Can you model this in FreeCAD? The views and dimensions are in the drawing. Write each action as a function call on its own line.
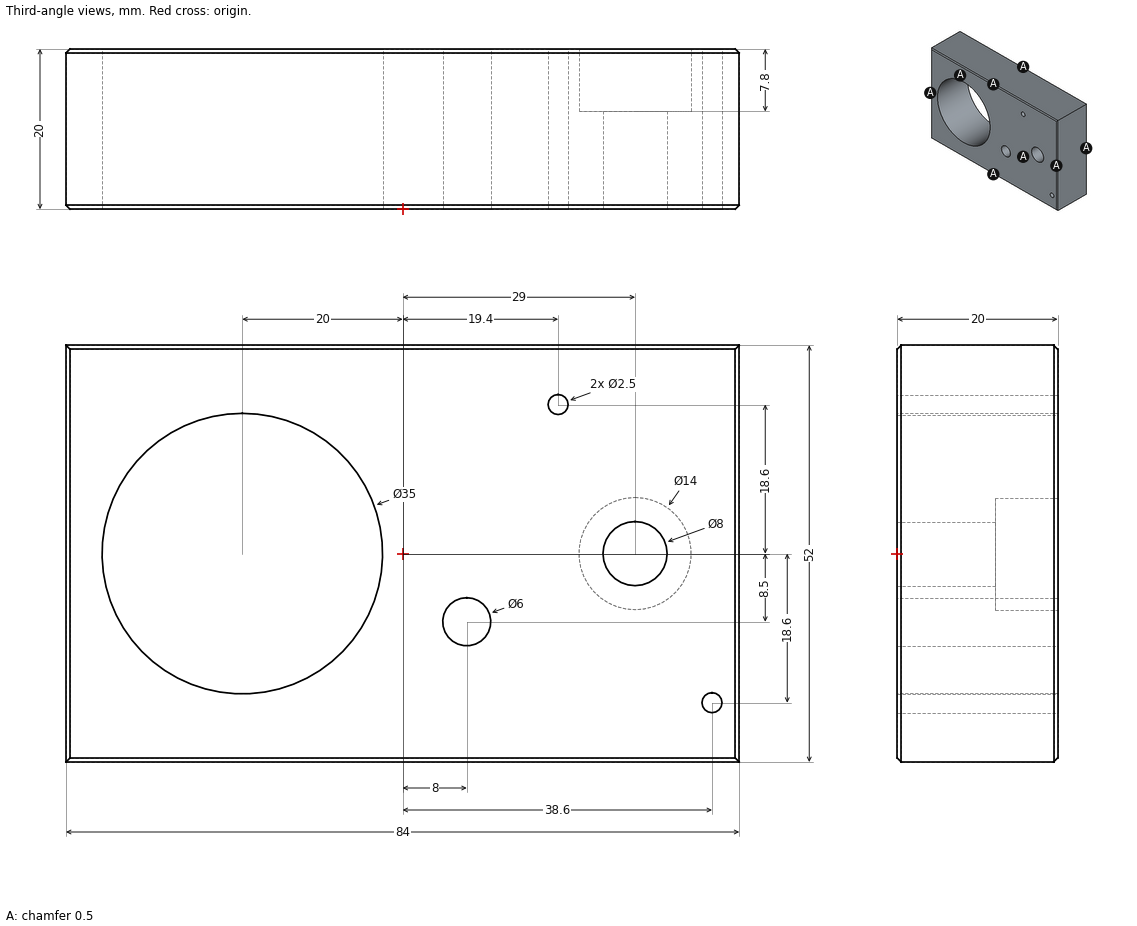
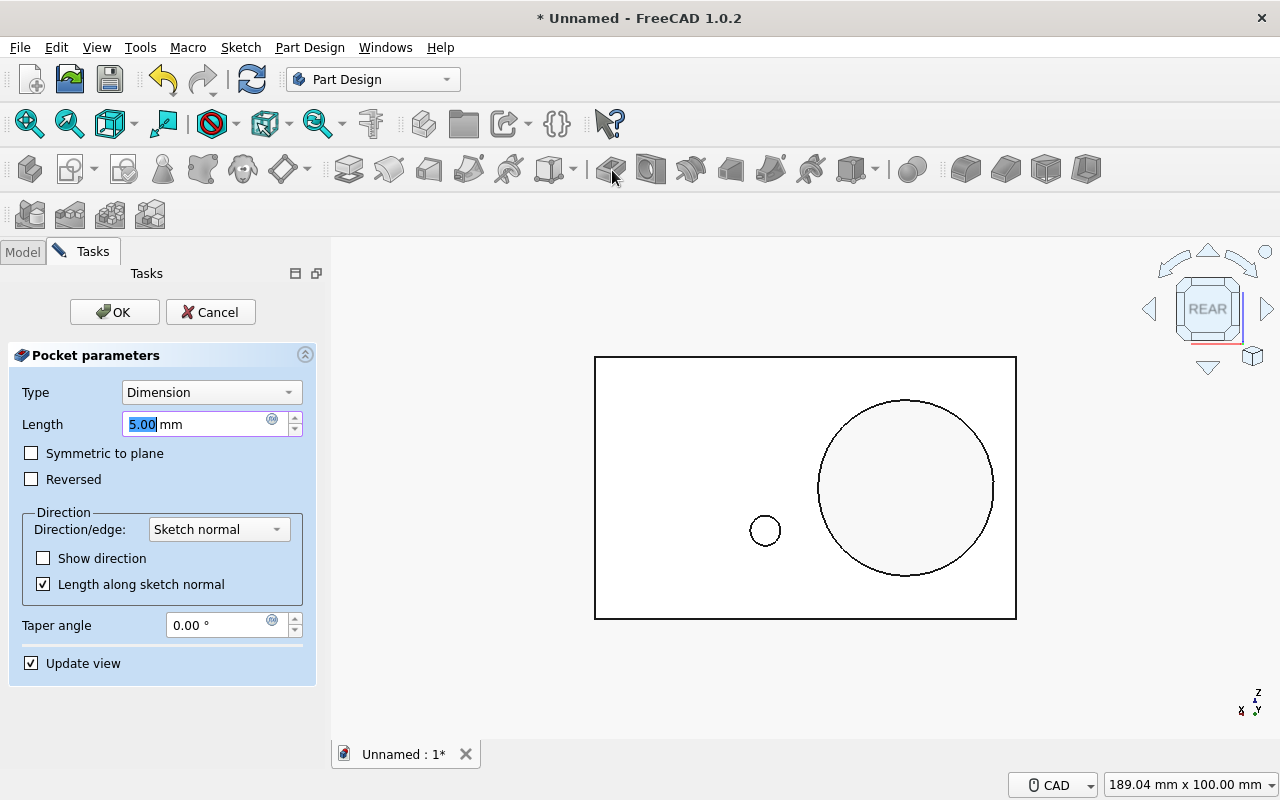
text(20)
key(Tab)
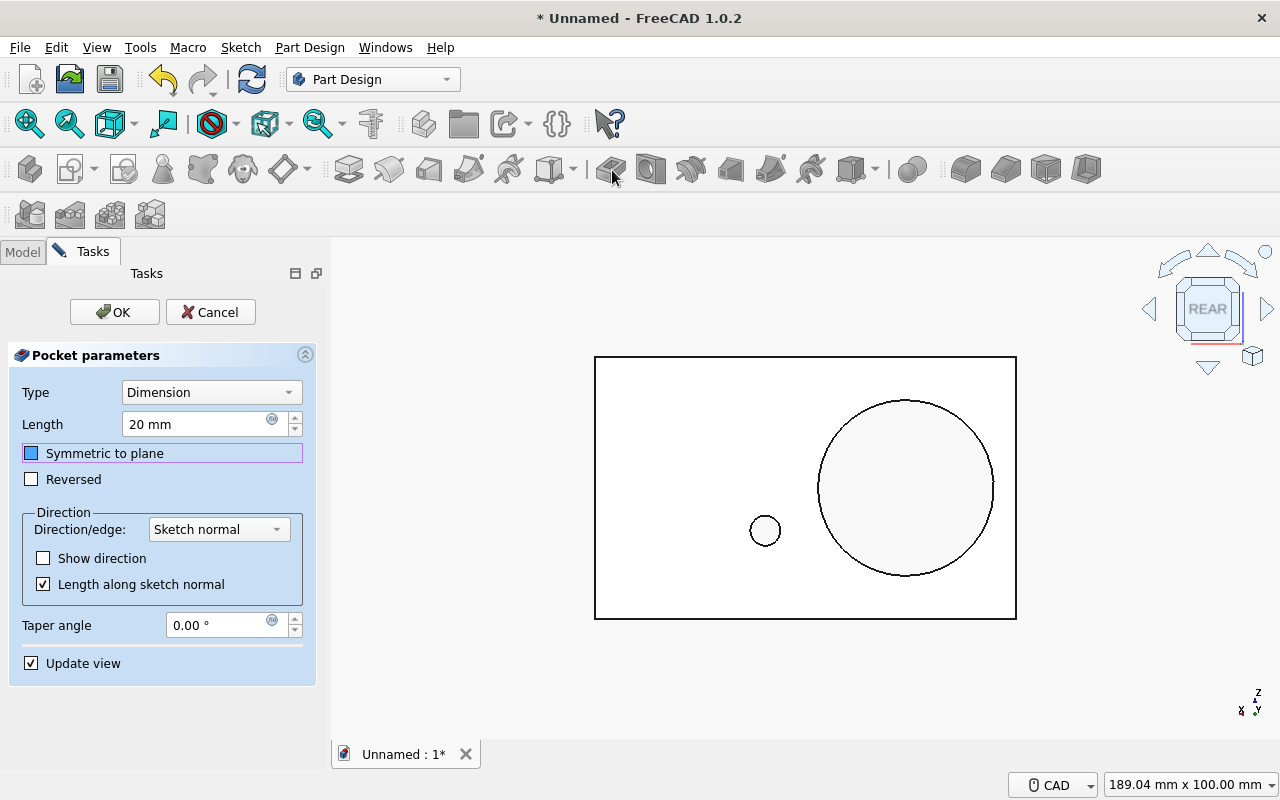
click(115, 312)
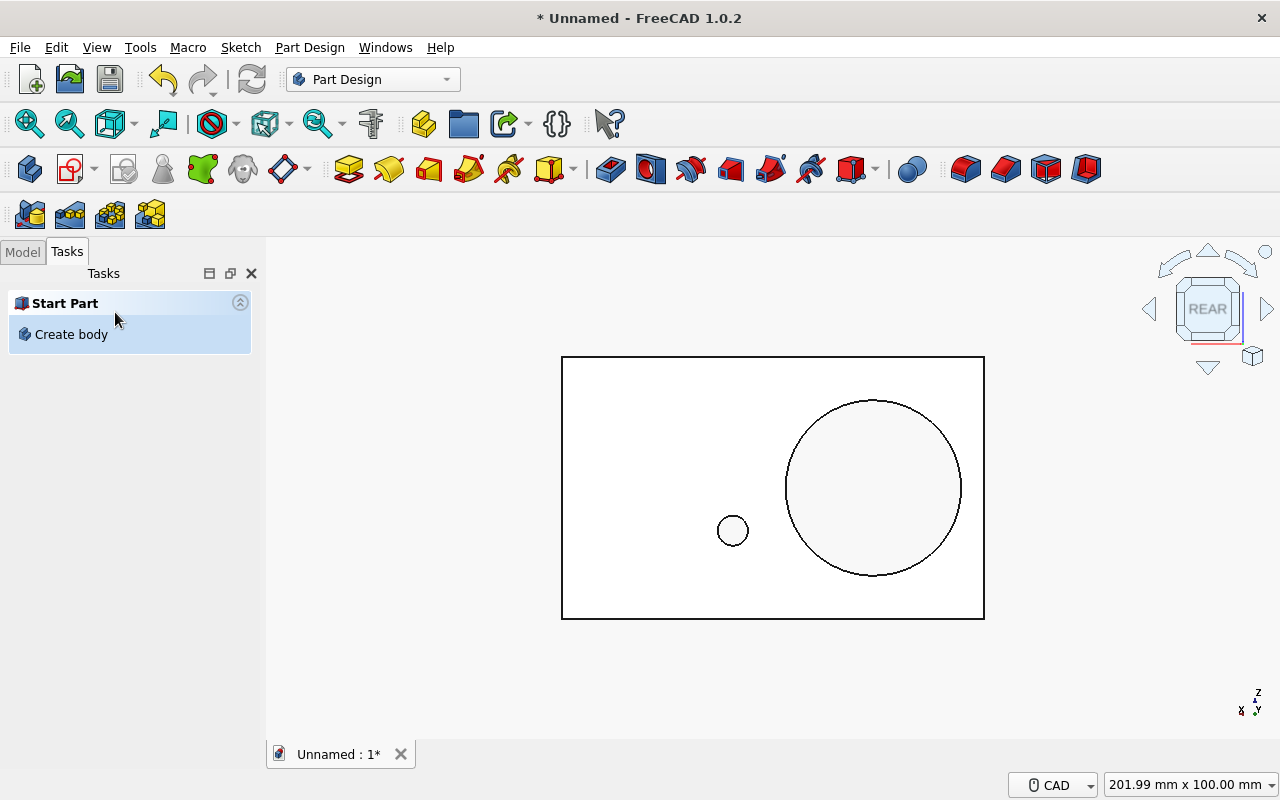
click(653, 450)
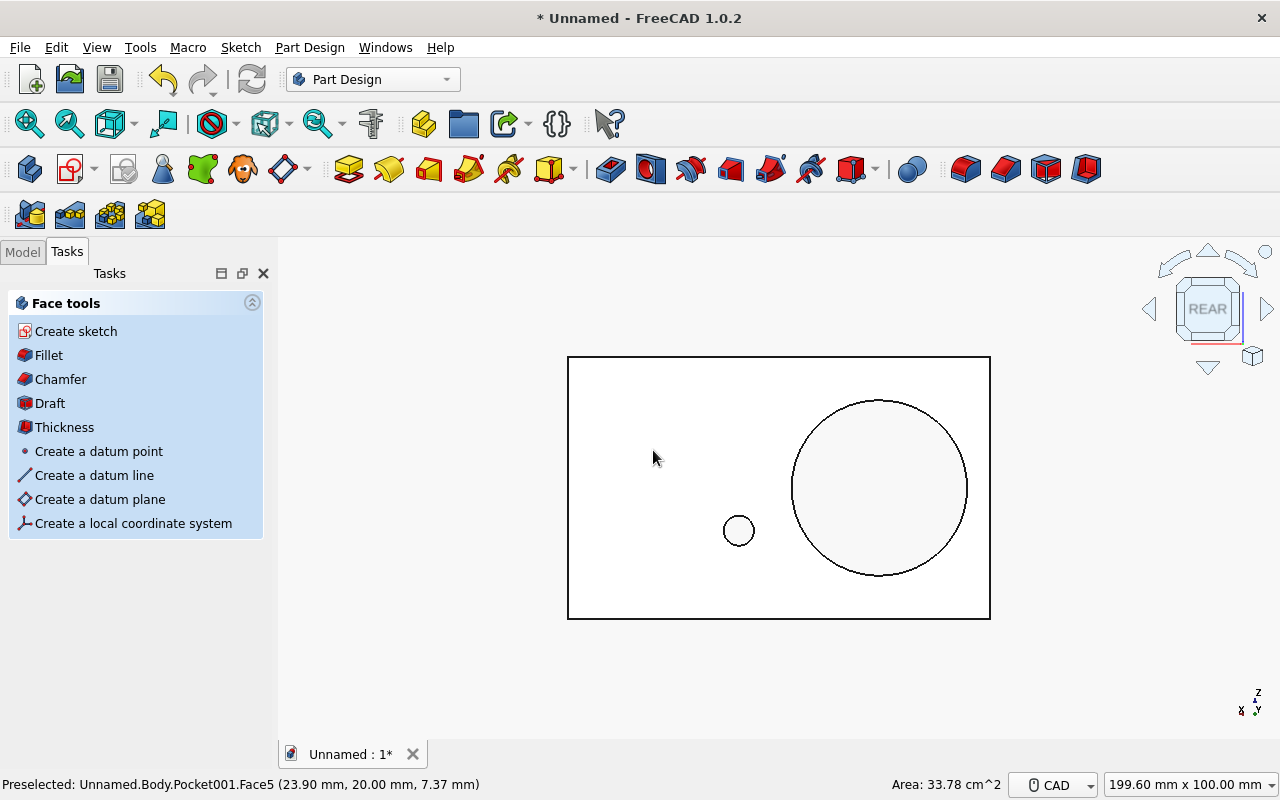
click(70, 170)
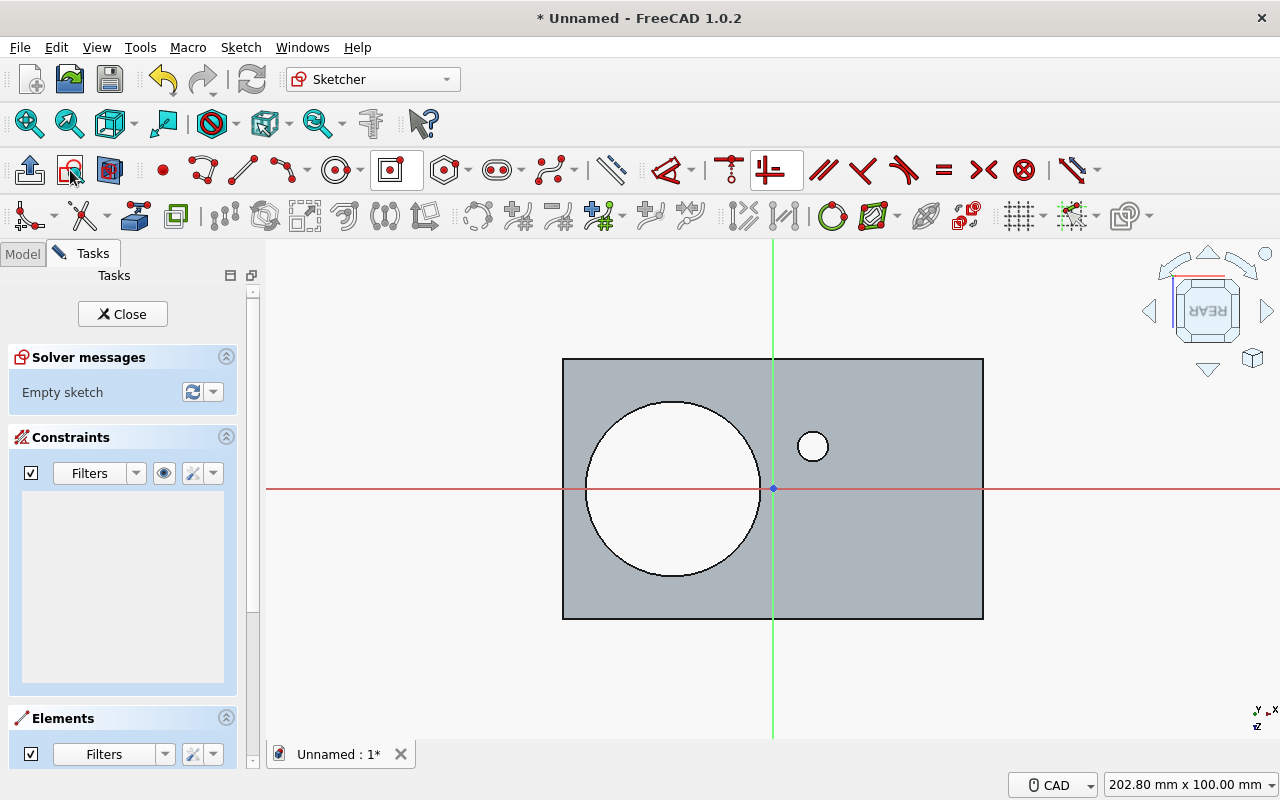
scroll(1115, 489, up, 2)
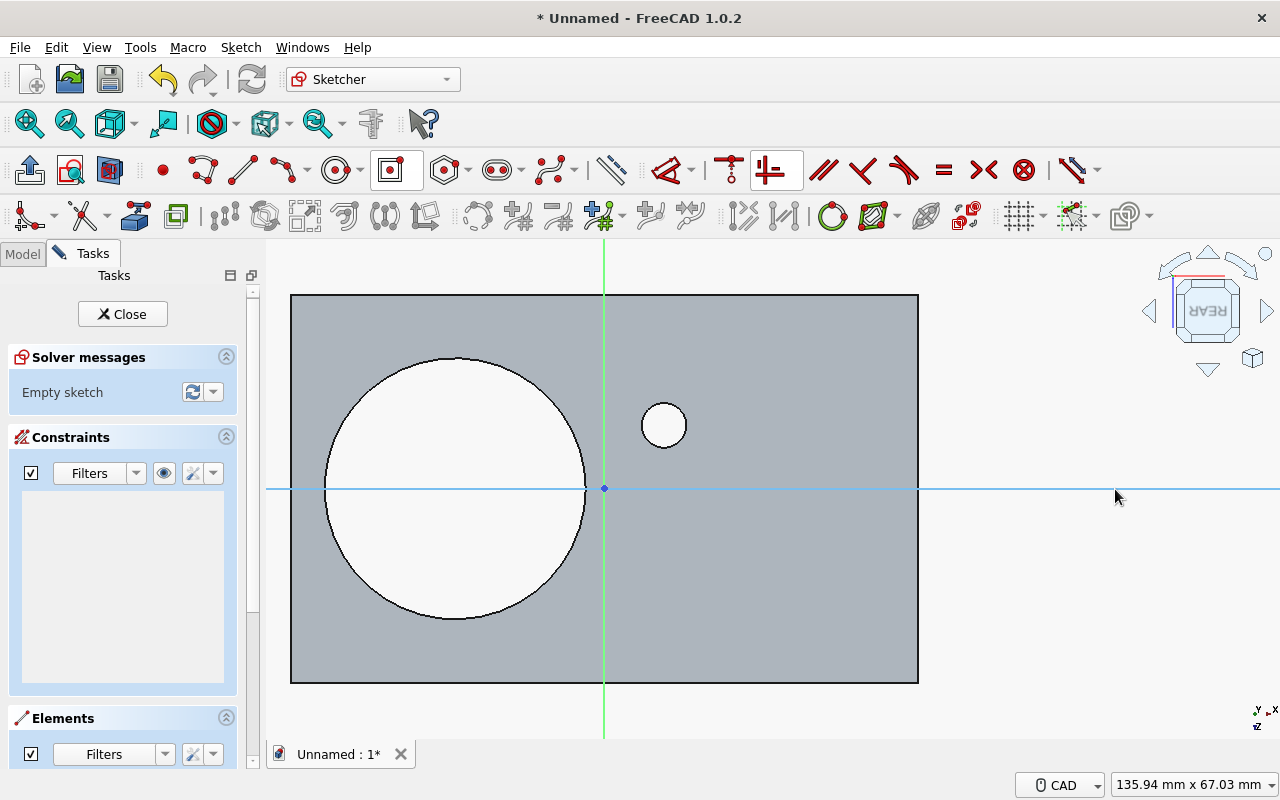
click(336, 170)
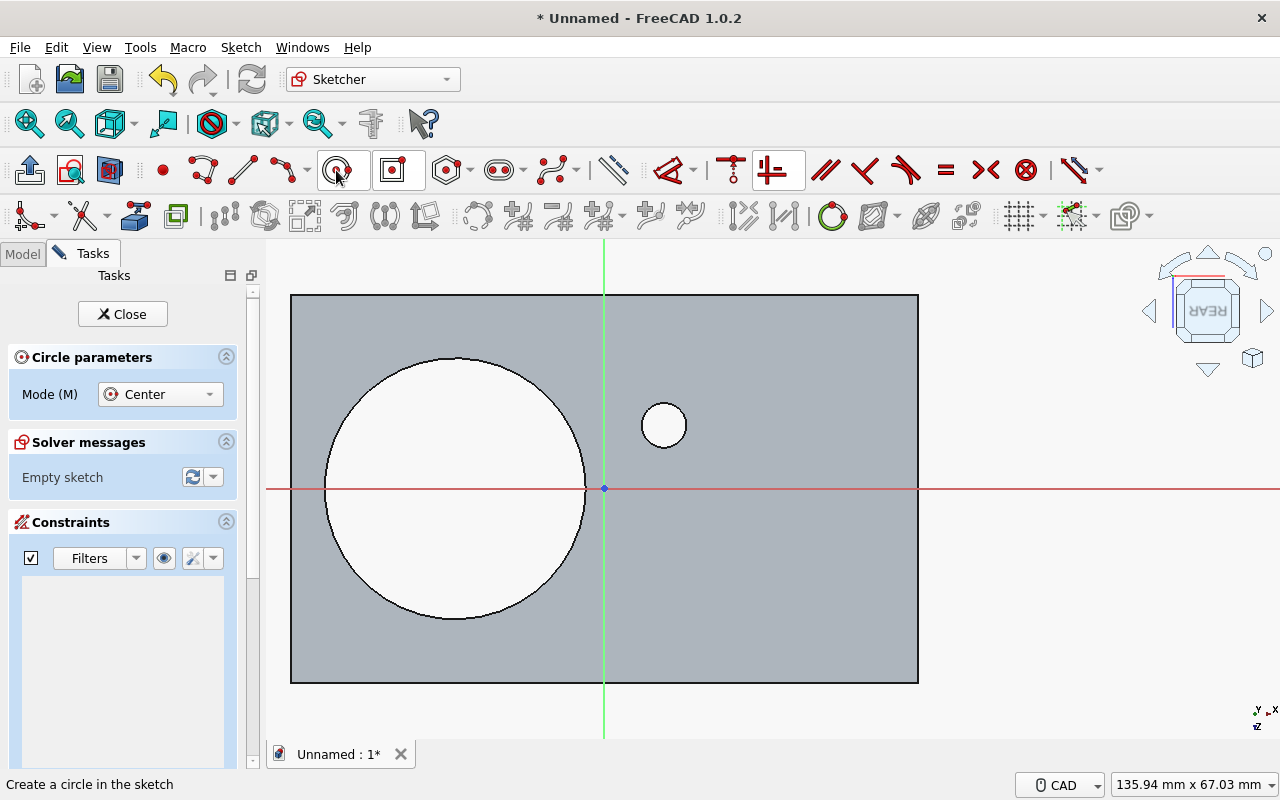
scroll(749, 627, up, 5)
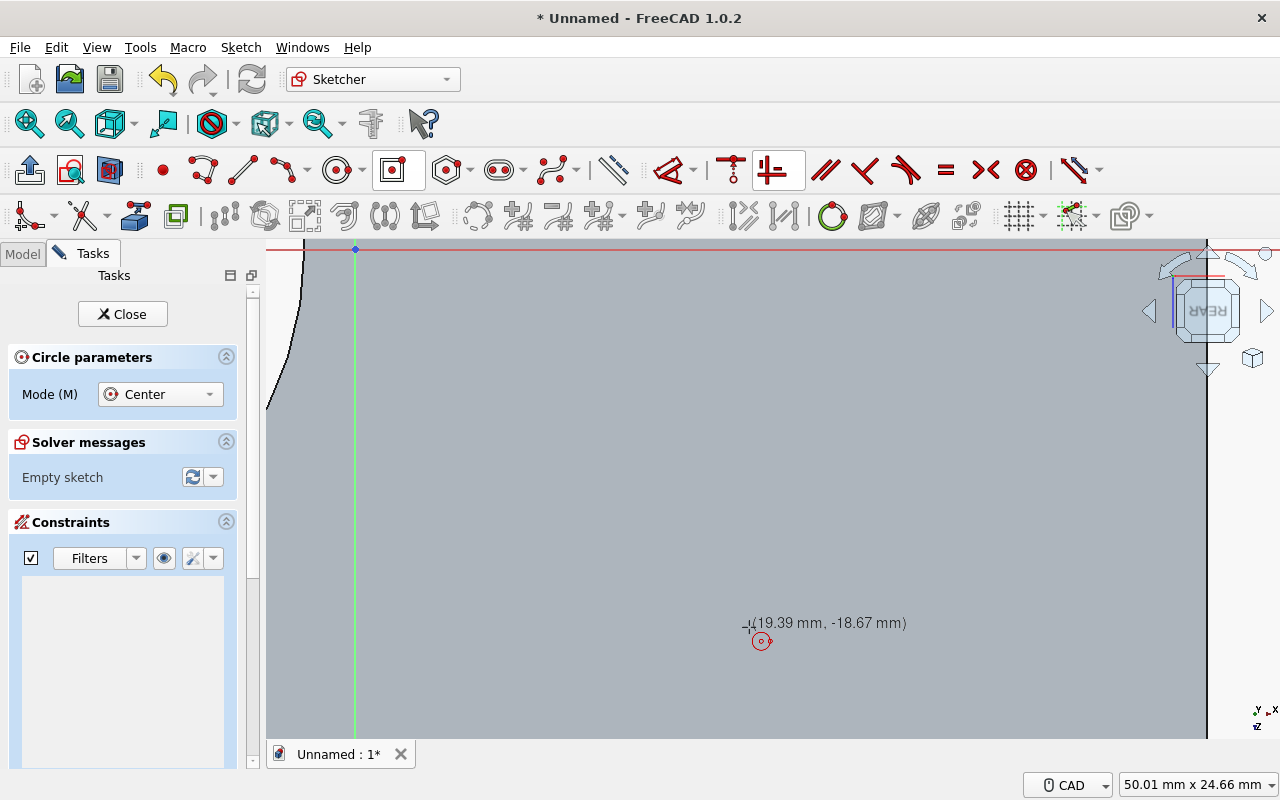
click(748, 627)
move(766, 609)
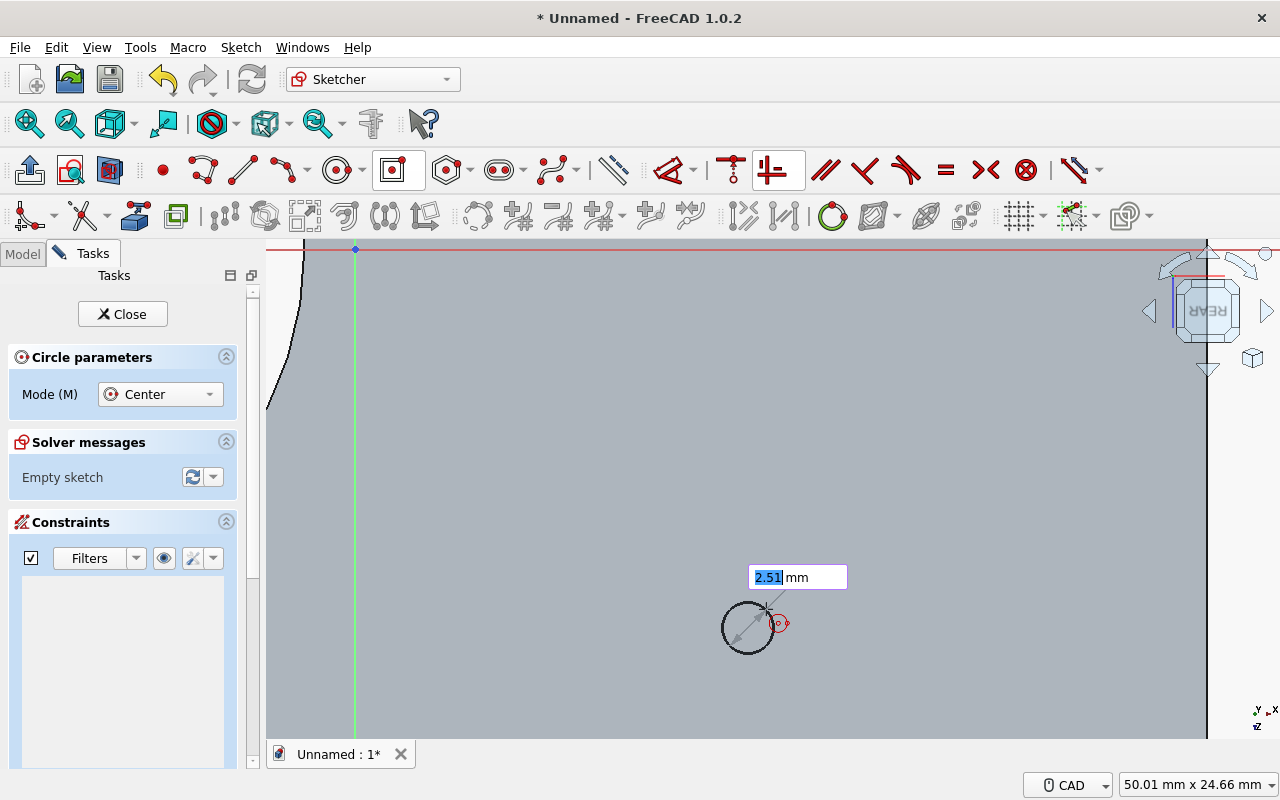
text(2.5)
key(Return)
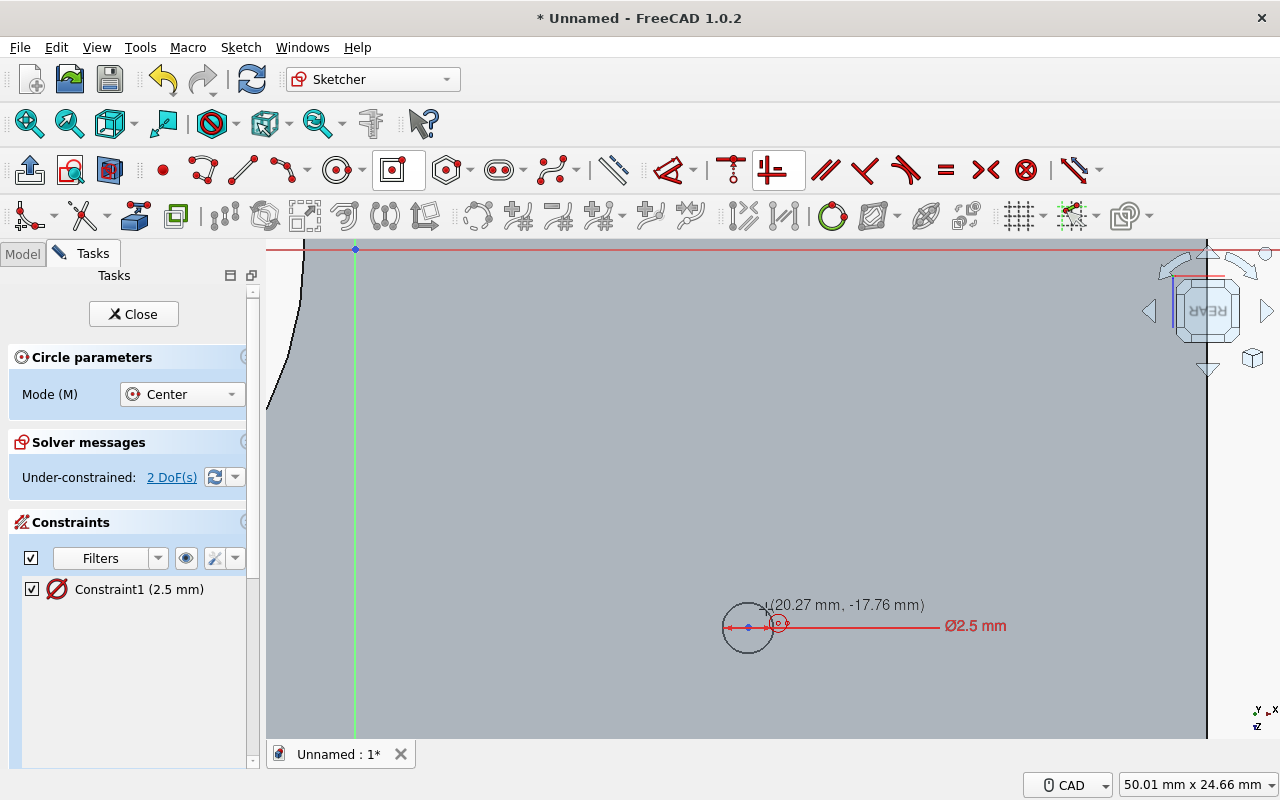
scroll(673, 628, down, 5)